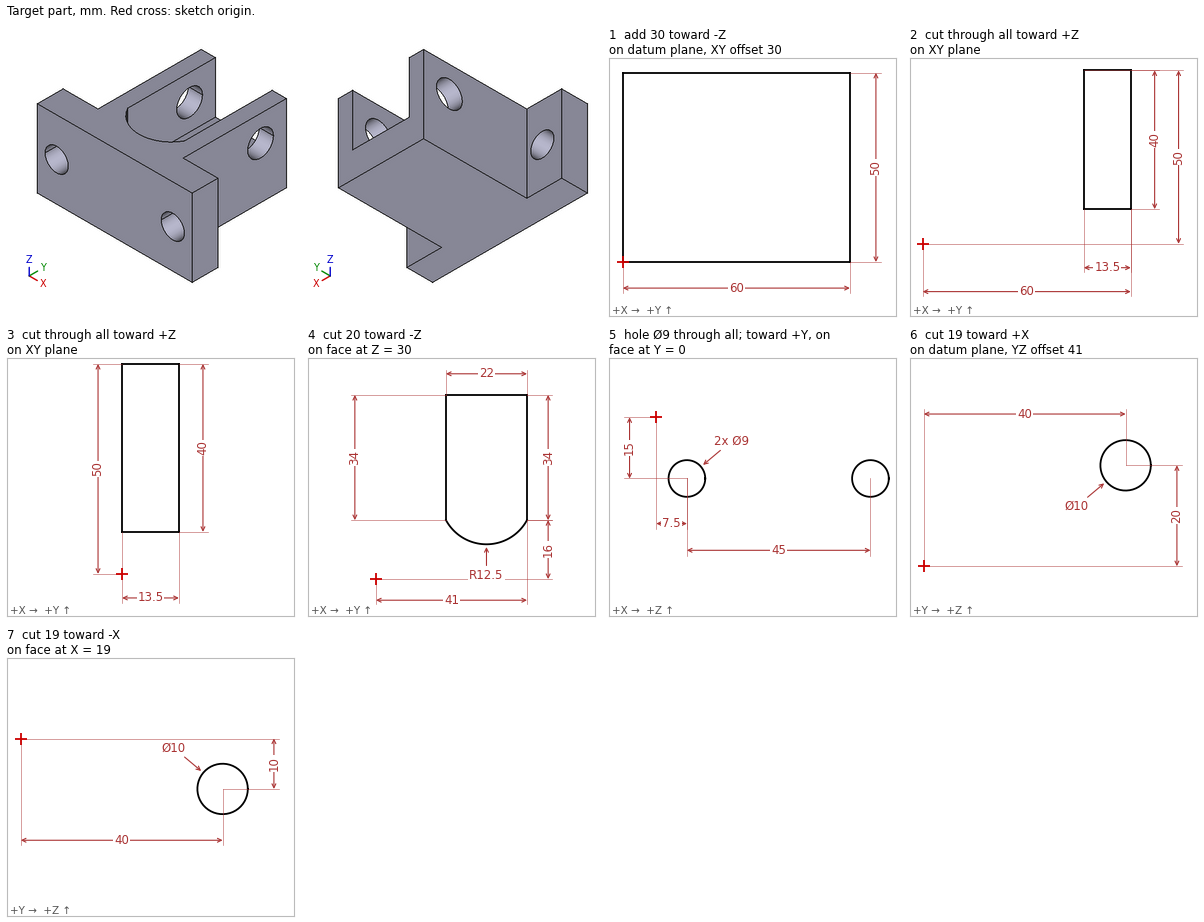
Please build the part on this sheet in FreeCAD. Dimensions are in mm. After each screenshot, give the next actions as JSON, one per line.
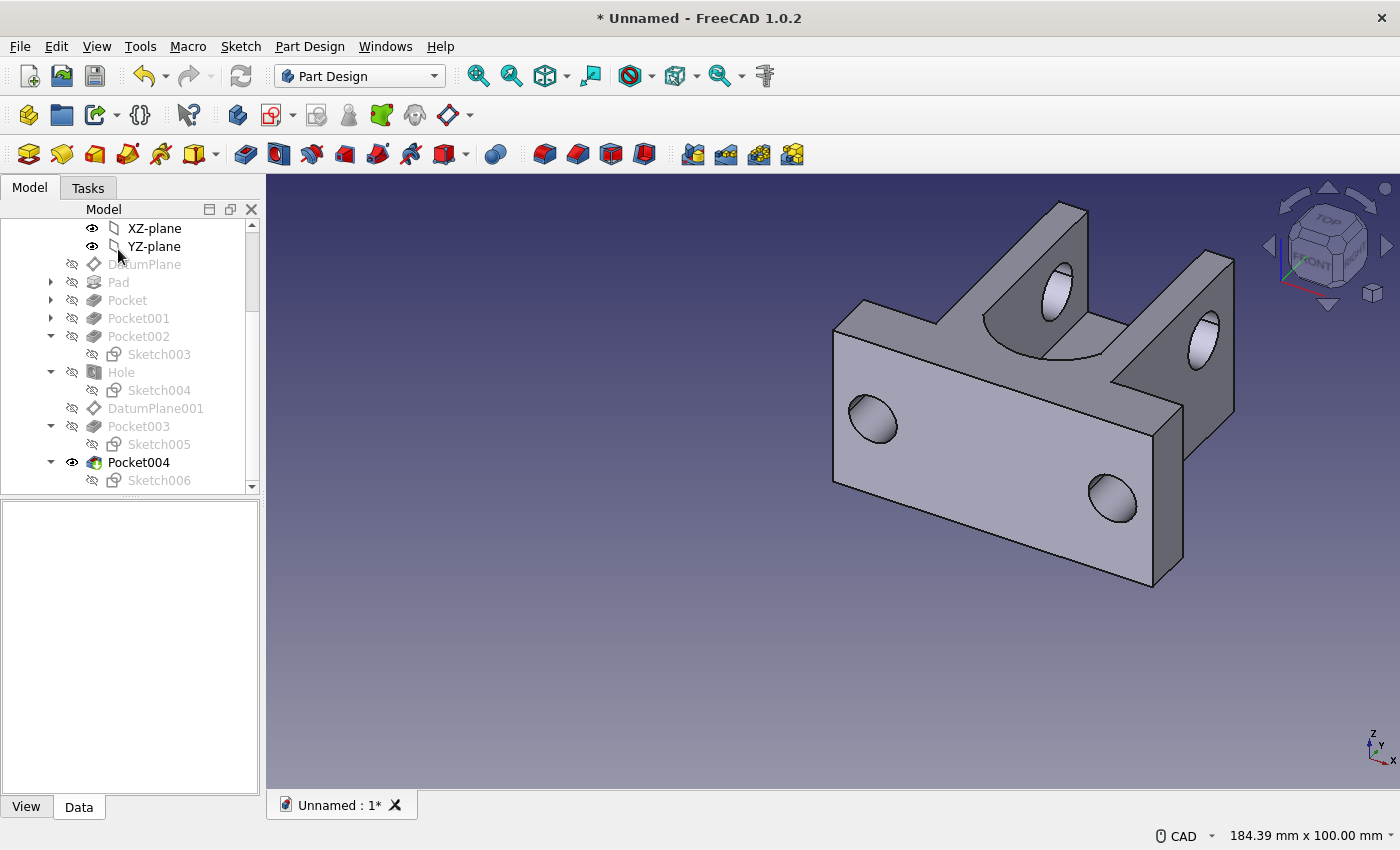
{"action": "key", "text": "0"}